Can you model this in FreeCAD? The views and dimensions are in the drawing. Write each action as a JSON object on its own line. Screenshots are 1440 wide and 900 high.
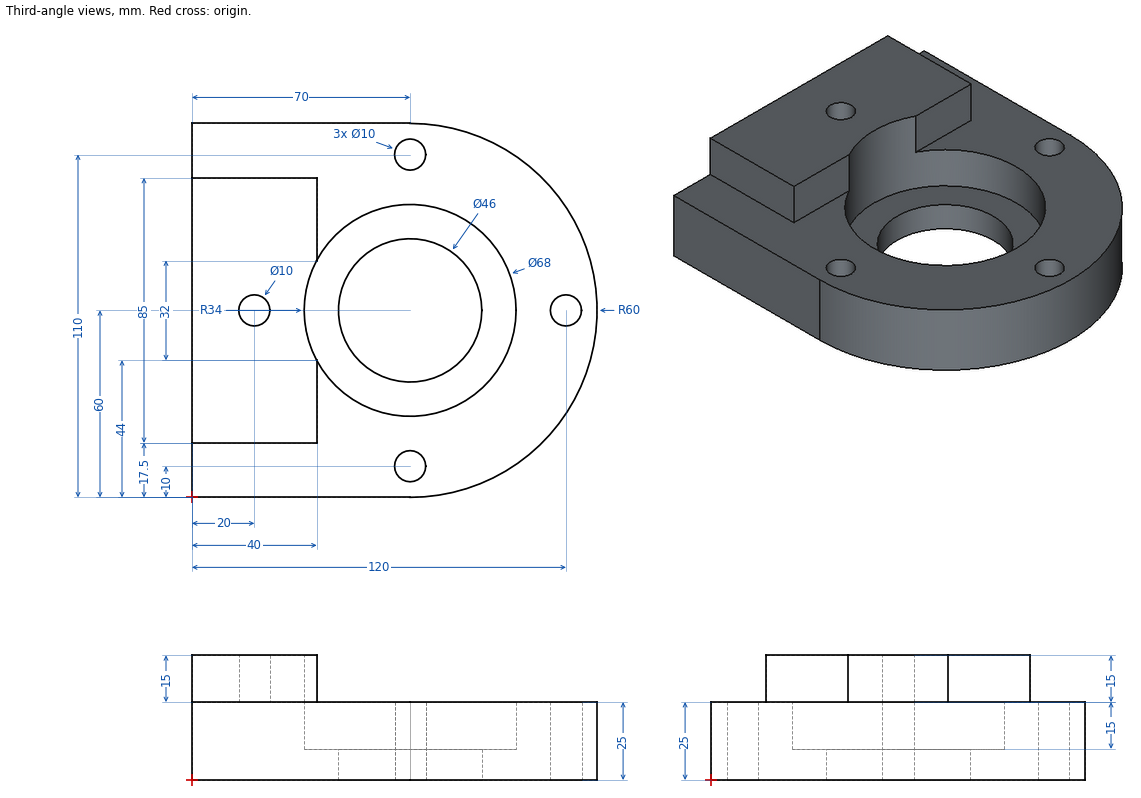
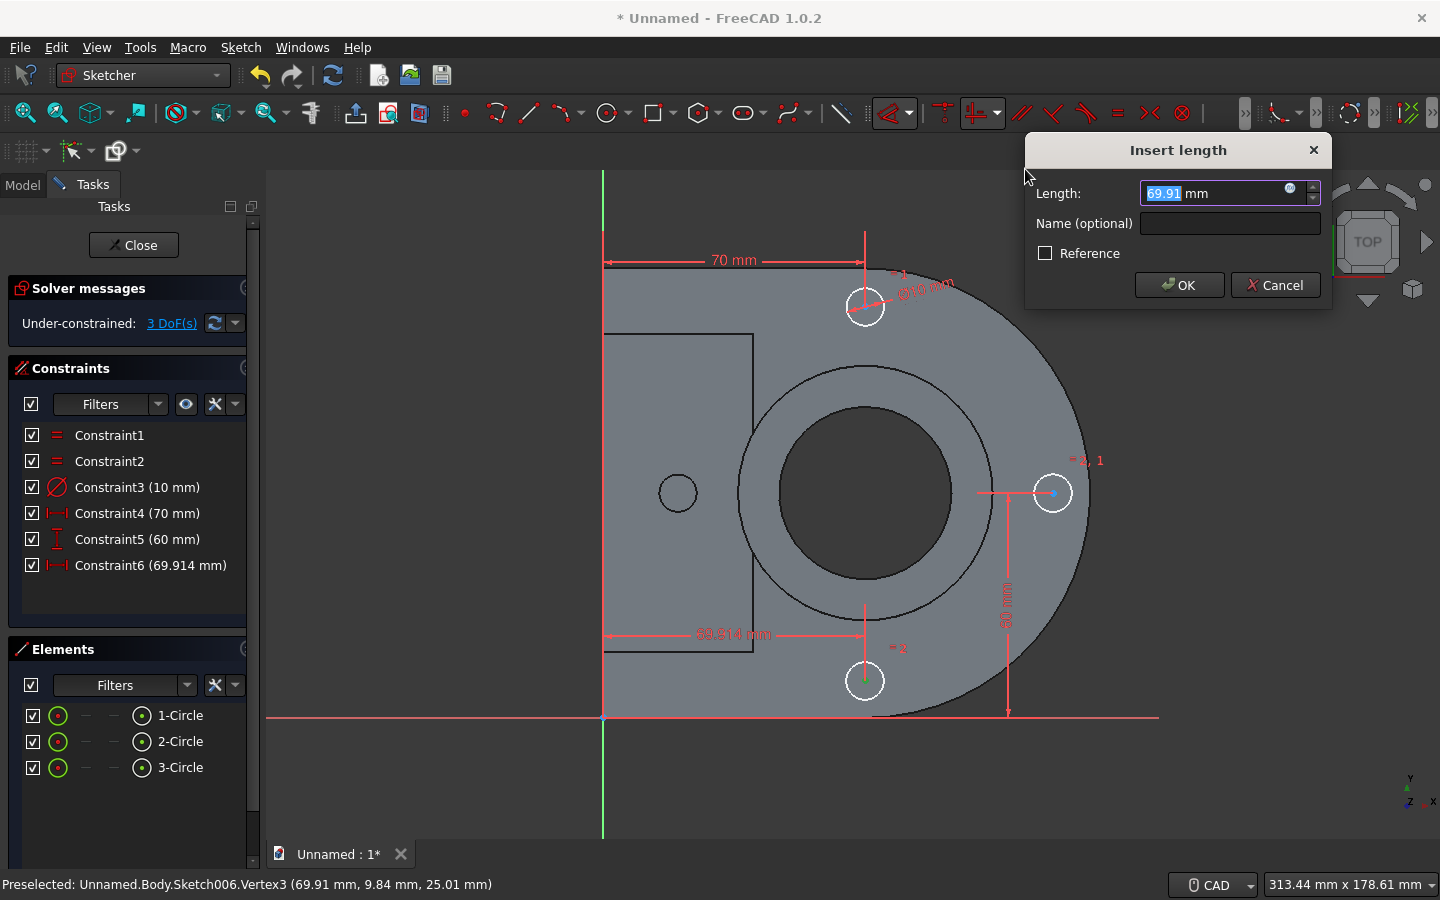
{"action": "type", "text": "70"}
{"action": "key", "text": "Return"}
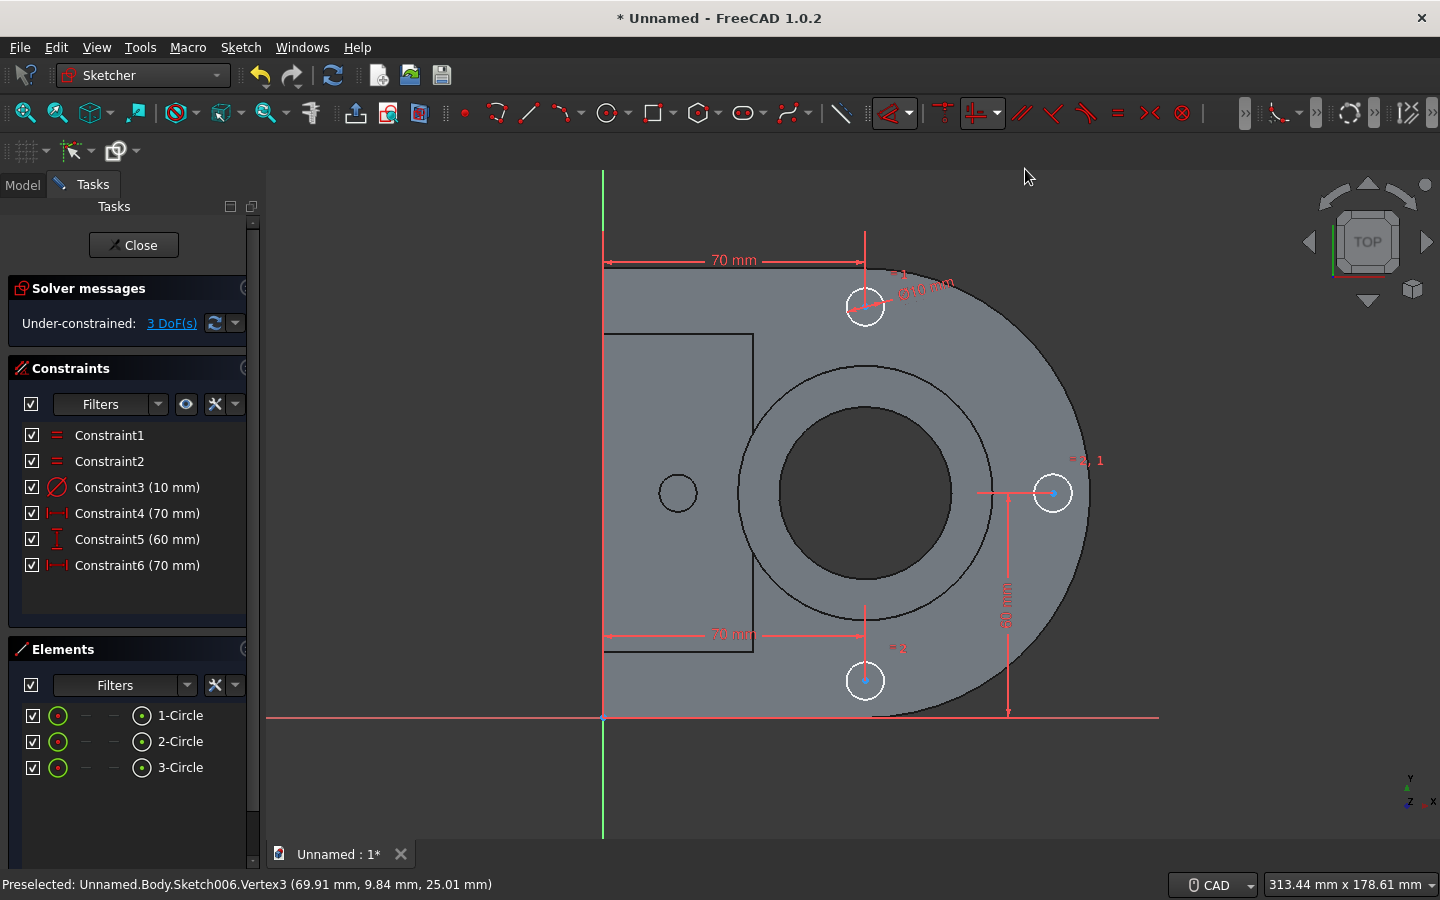
{"action": "left_click", "coordinate": [865, 681]}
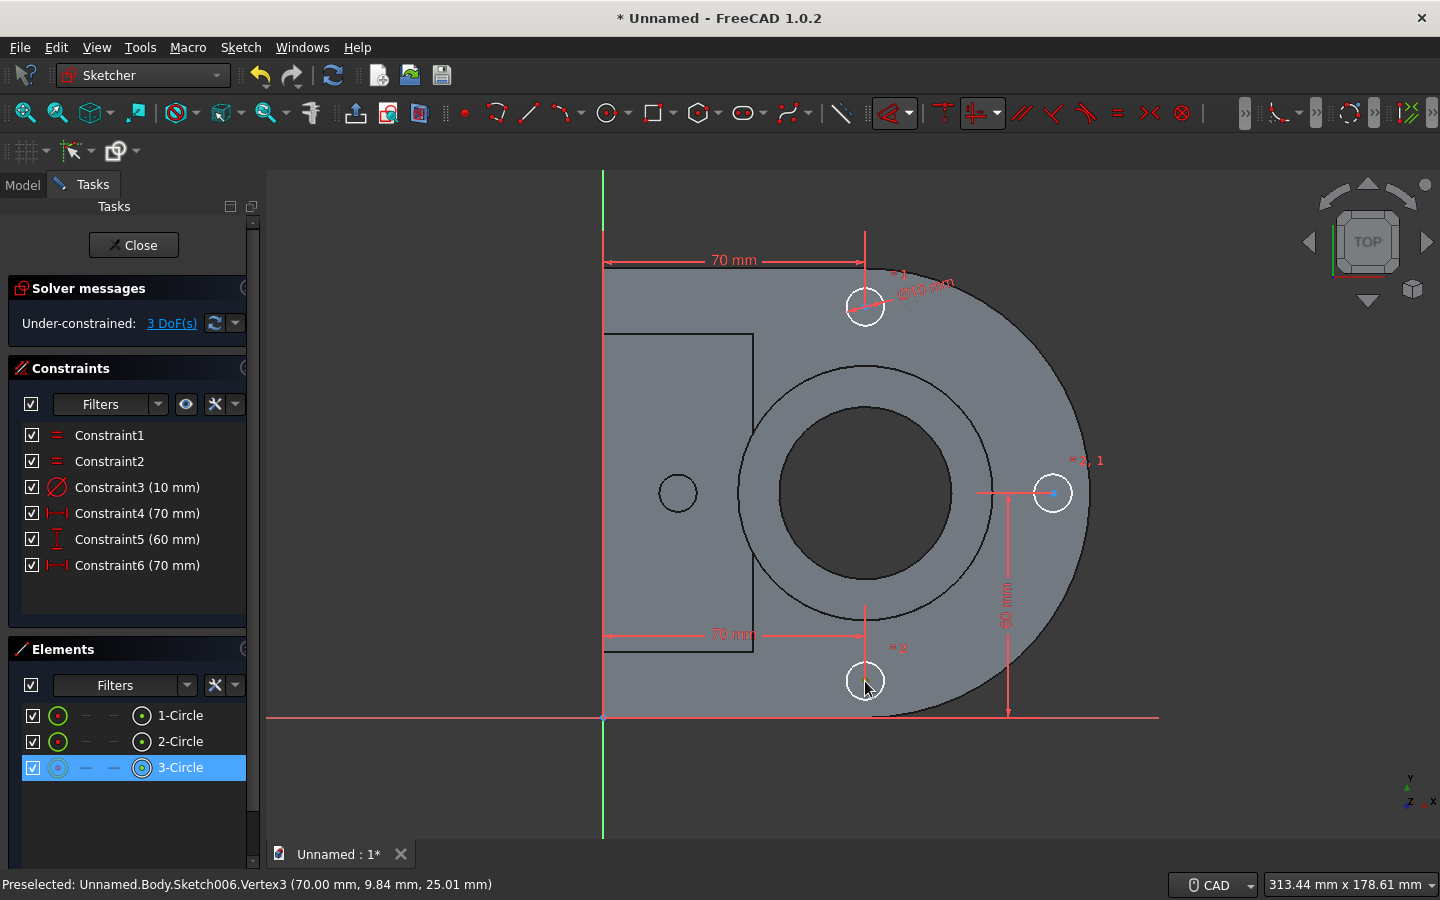
{"action": "key", "text": "i"}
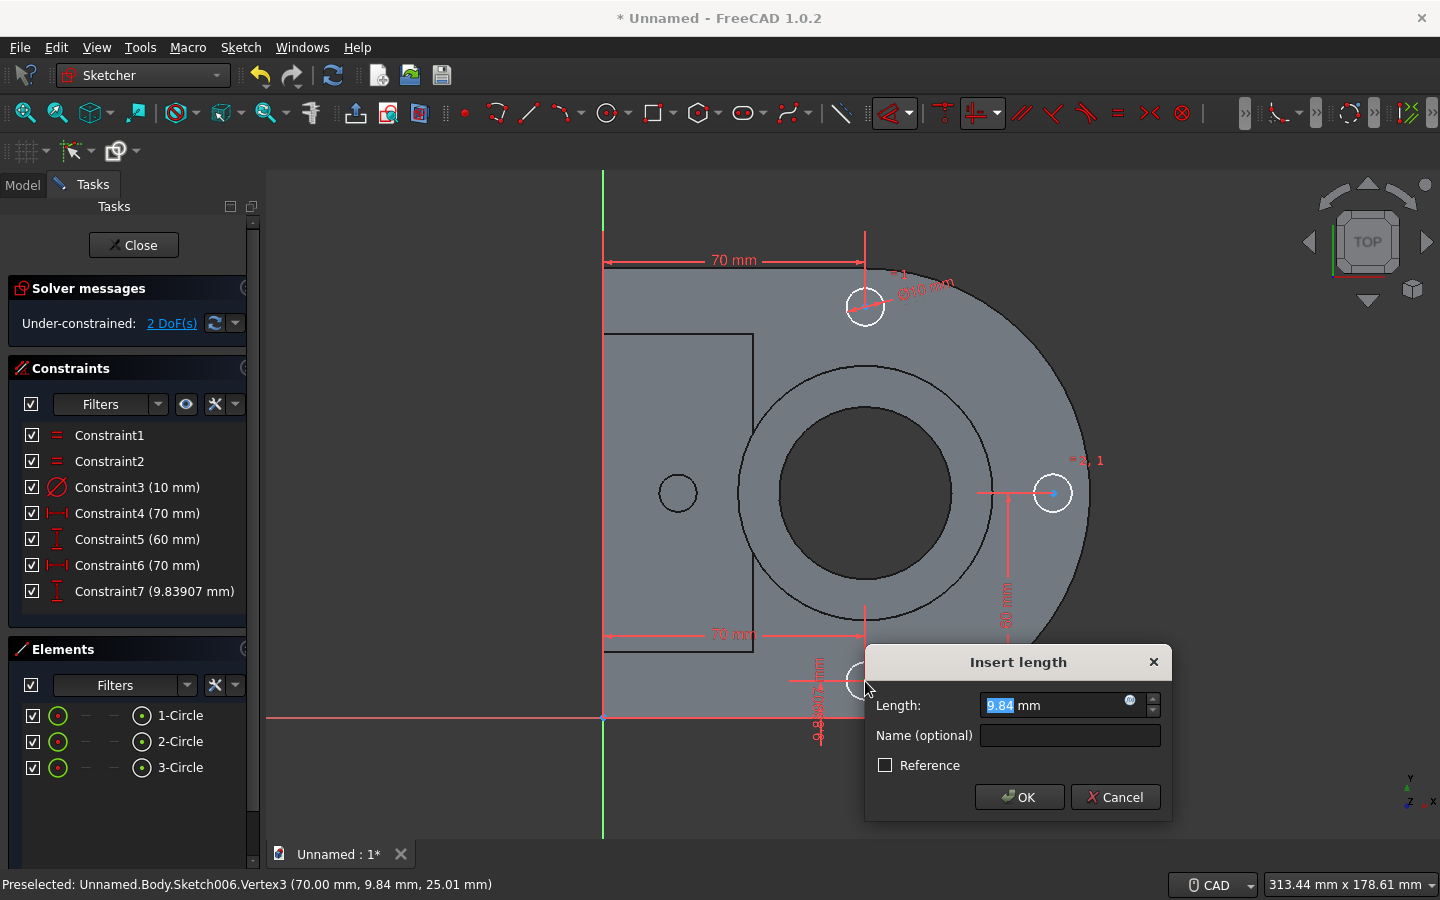
{"action": "type", "text": "10"}
{"action": "key", "text": "Return"}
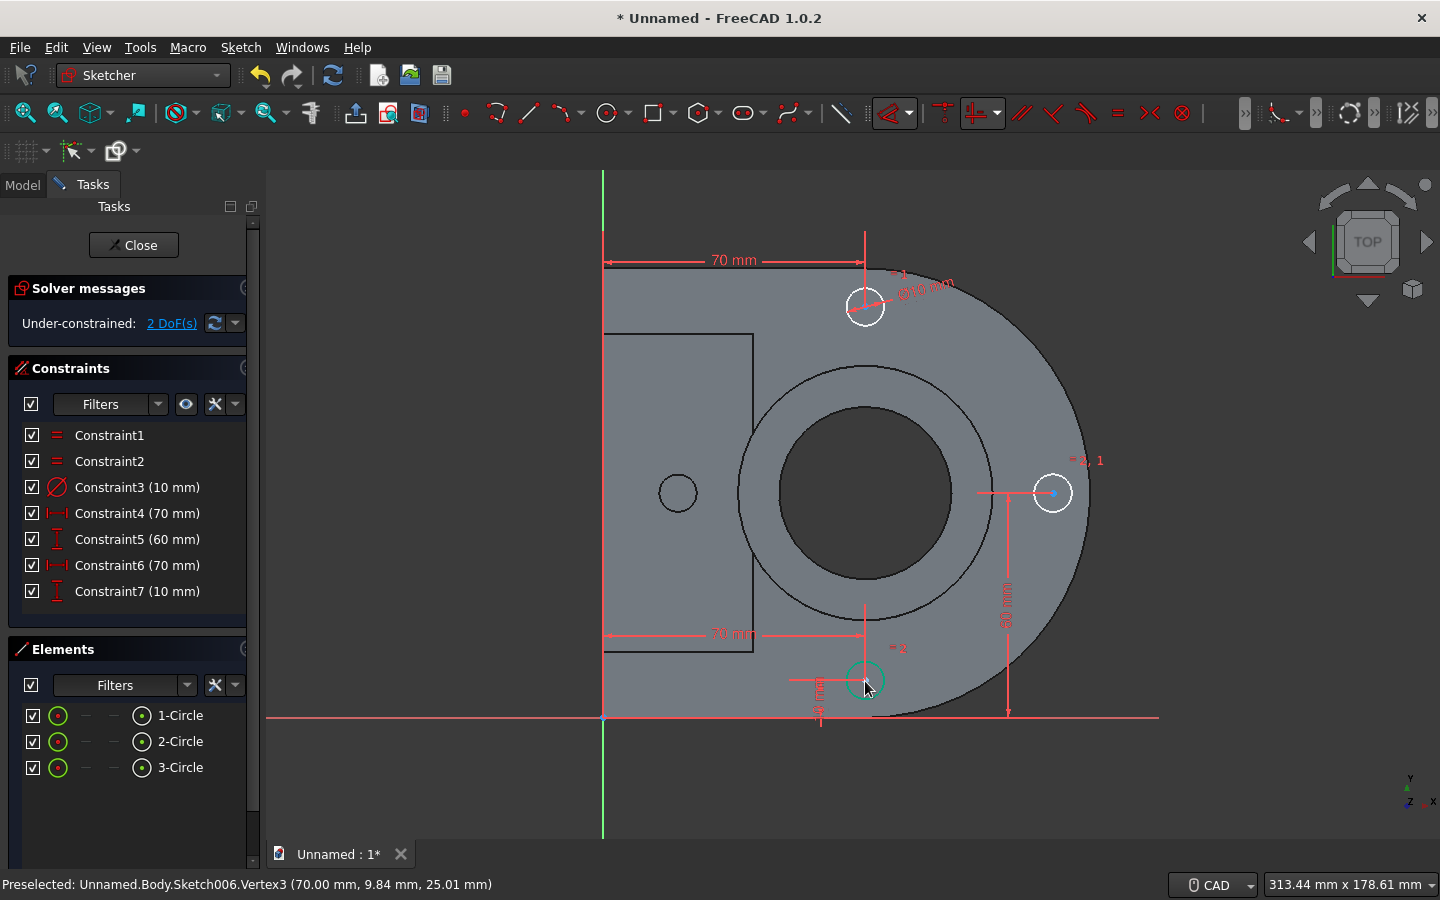
{"action": "left_click", "coordinate": [865, 307]}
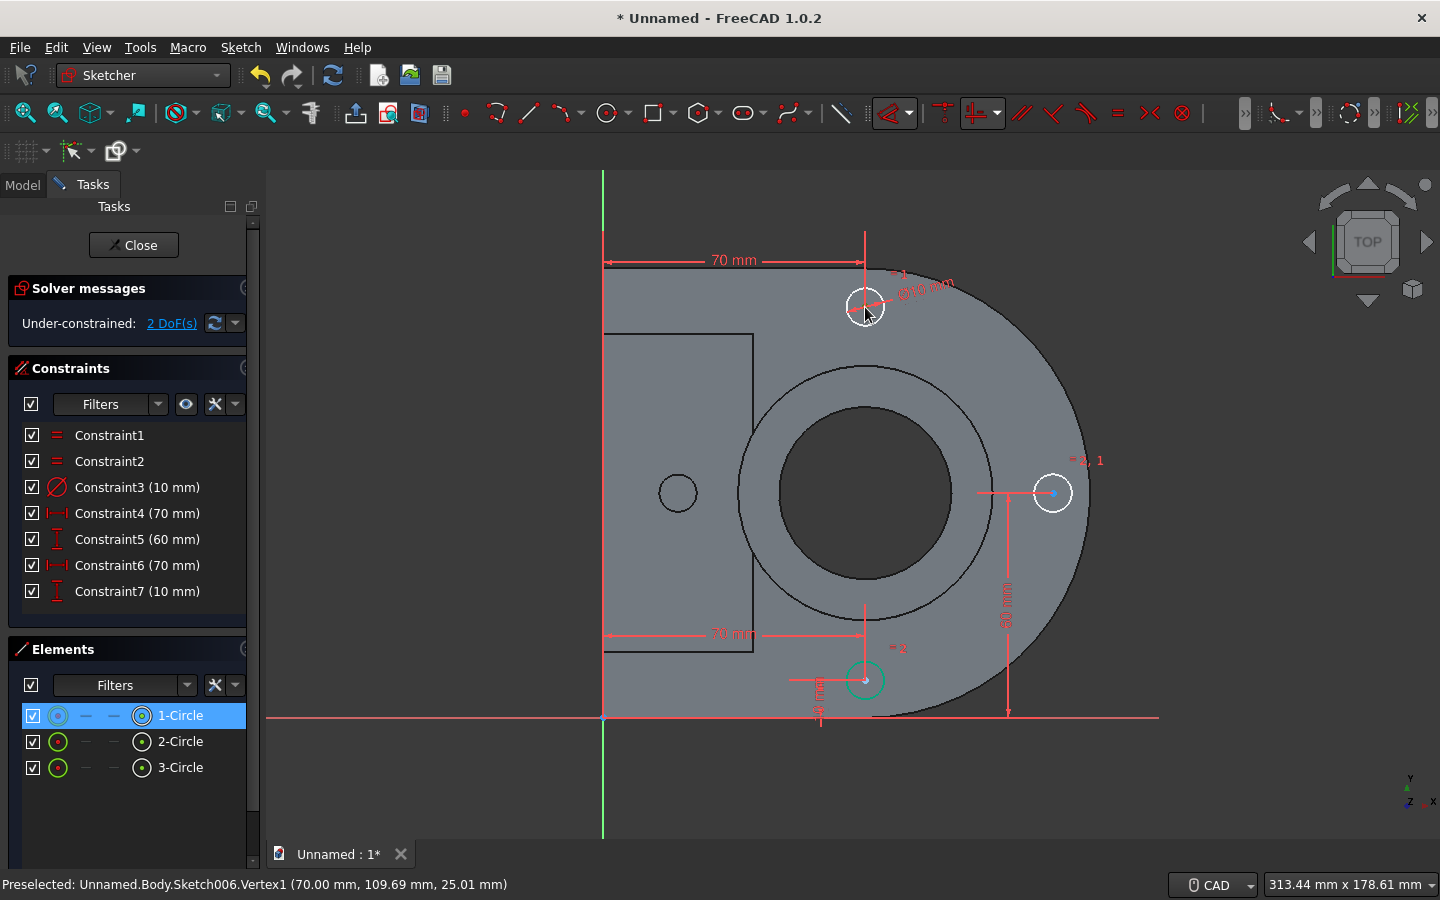
{"action": "key", "text": "i"}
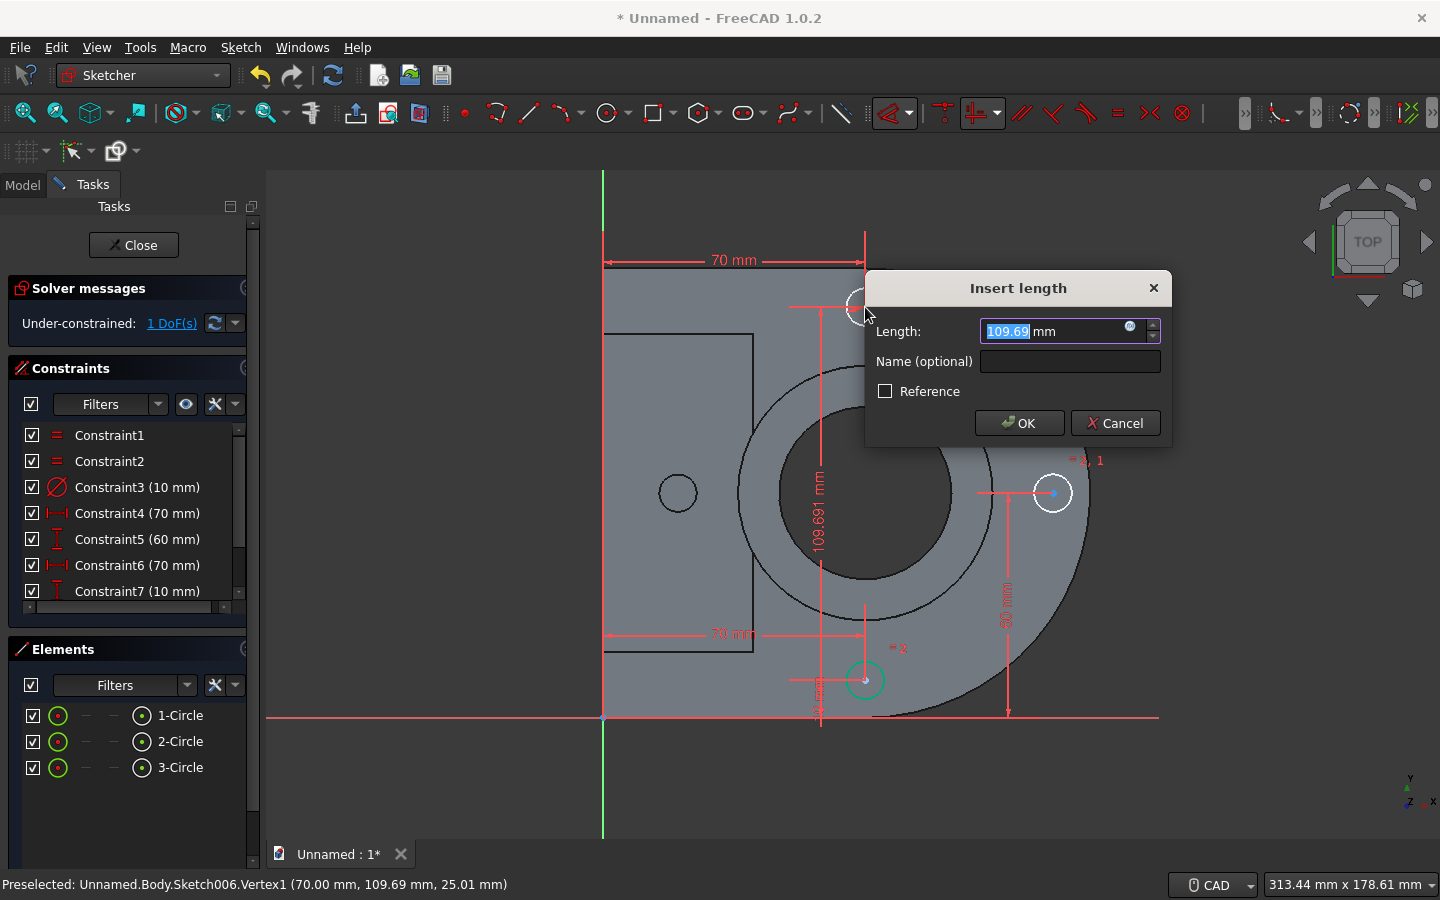
{"action": "type", "text": "110"}
{"action": "key", "text": "Return"}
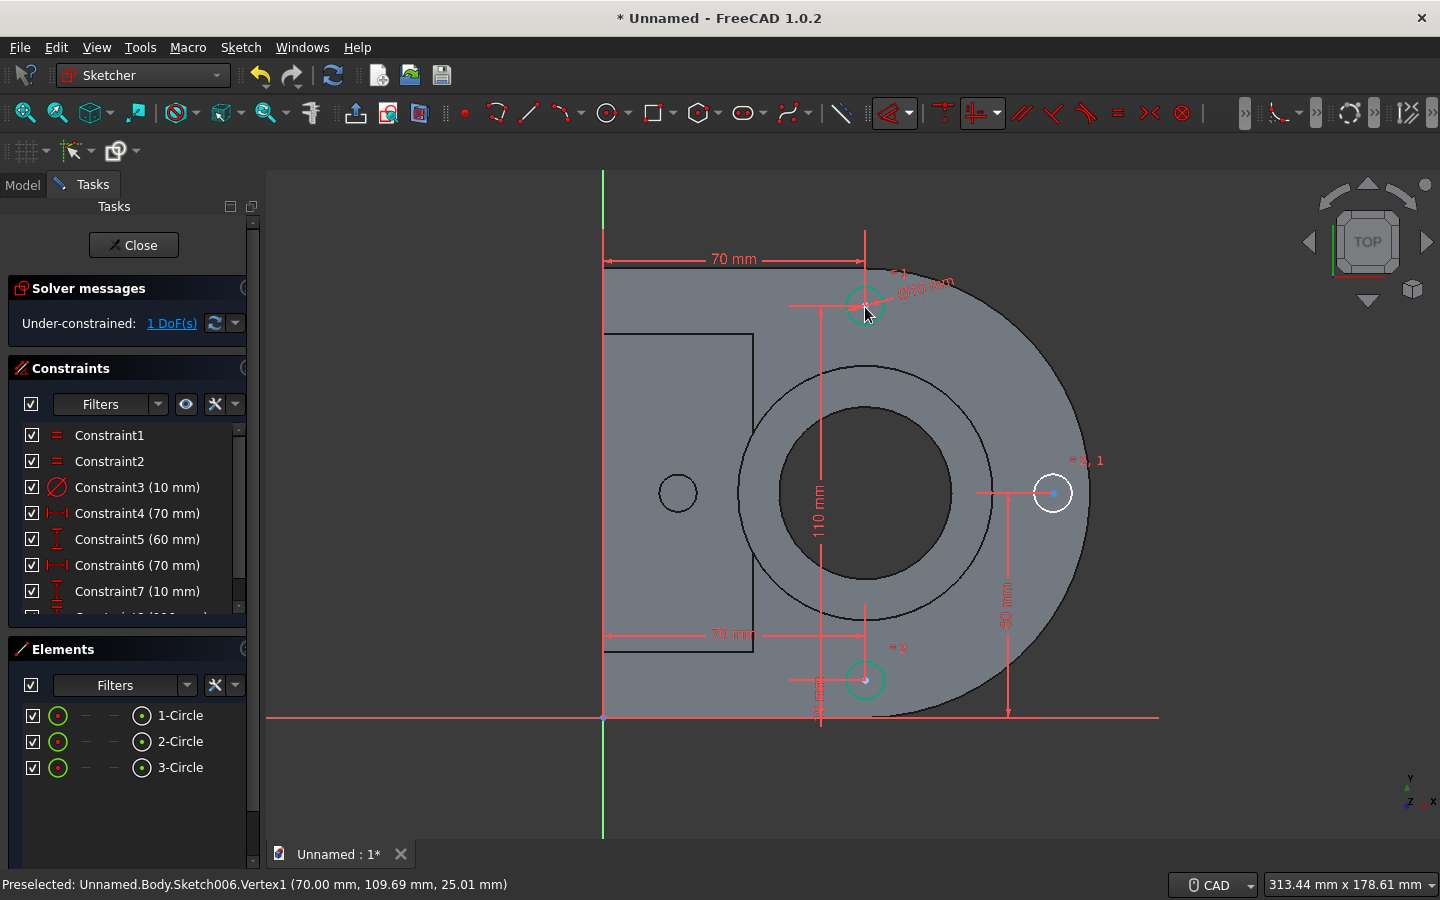
{"action": "left_click", "coordinate": [1053, 493]}